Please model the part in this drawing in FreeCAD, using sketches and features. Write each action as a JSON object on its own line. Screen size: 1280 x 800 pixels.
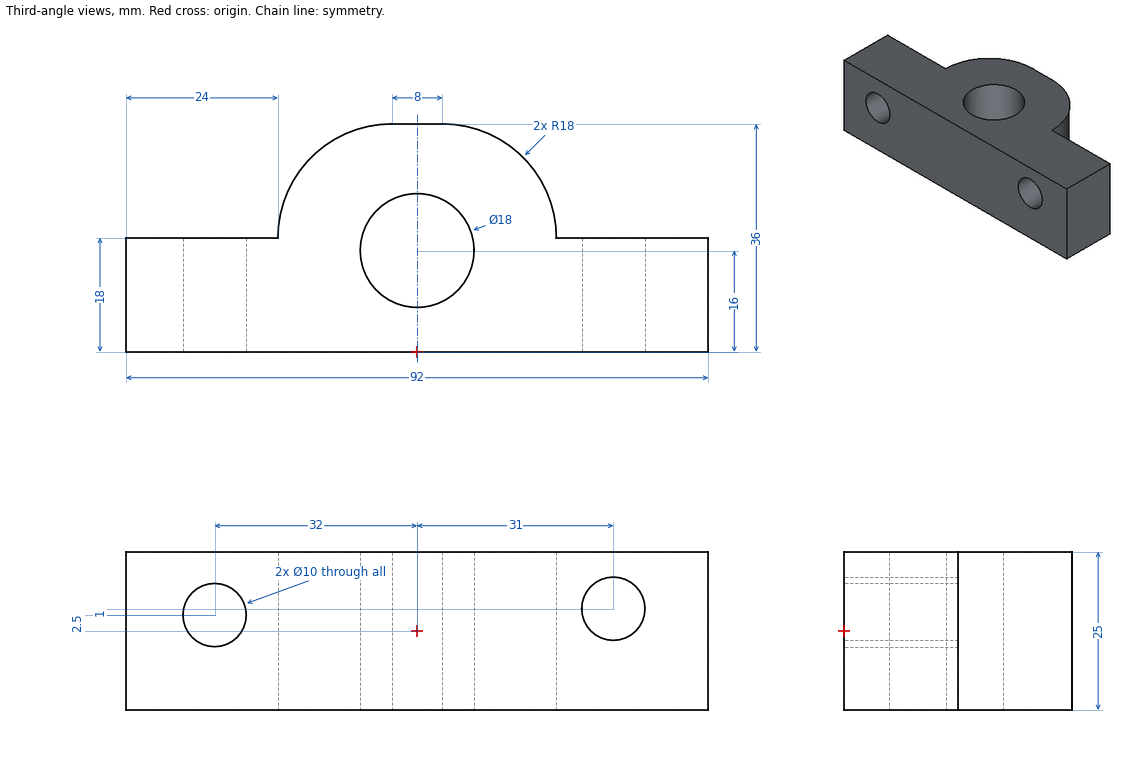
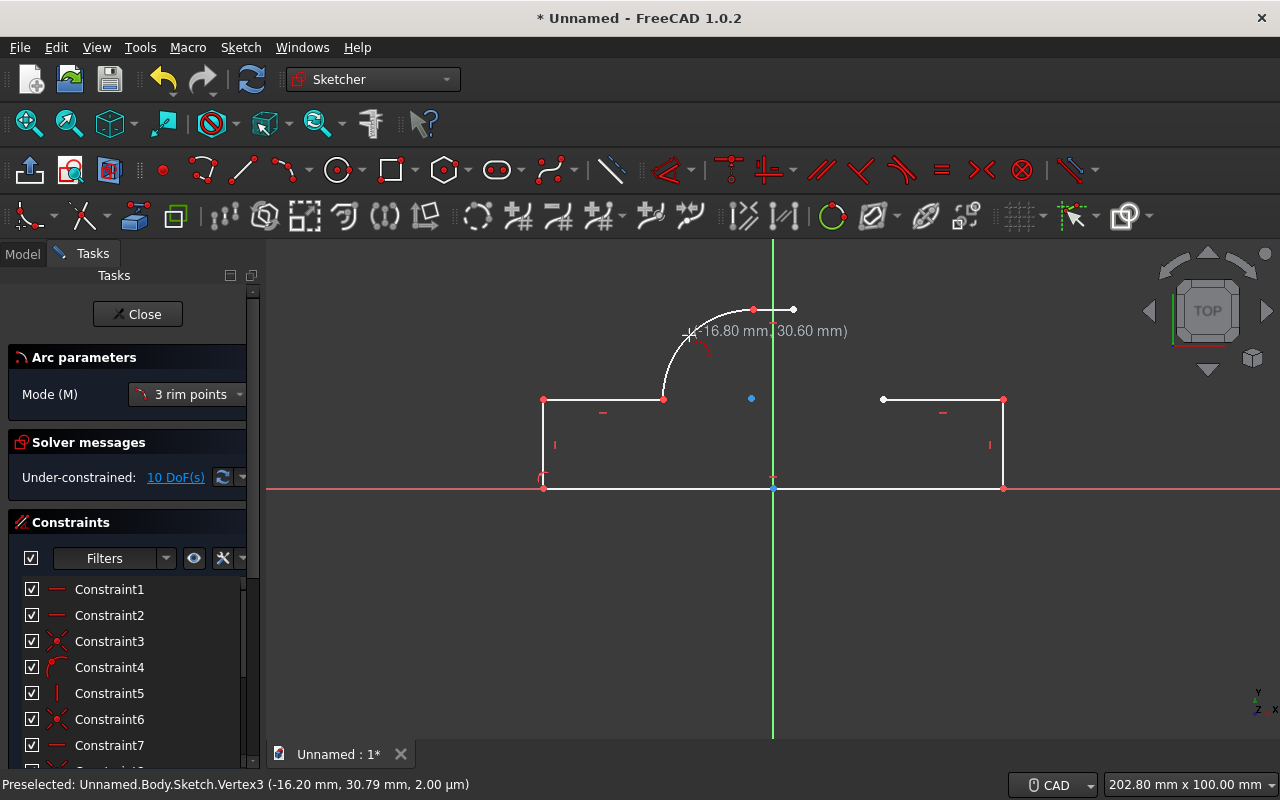
{"action": "left_click", "coordinate": [883, 400]}
{"action": "left_click", "coordinate": [793, 310]}
{"action": "left_click", "coordinate": [857, 335]}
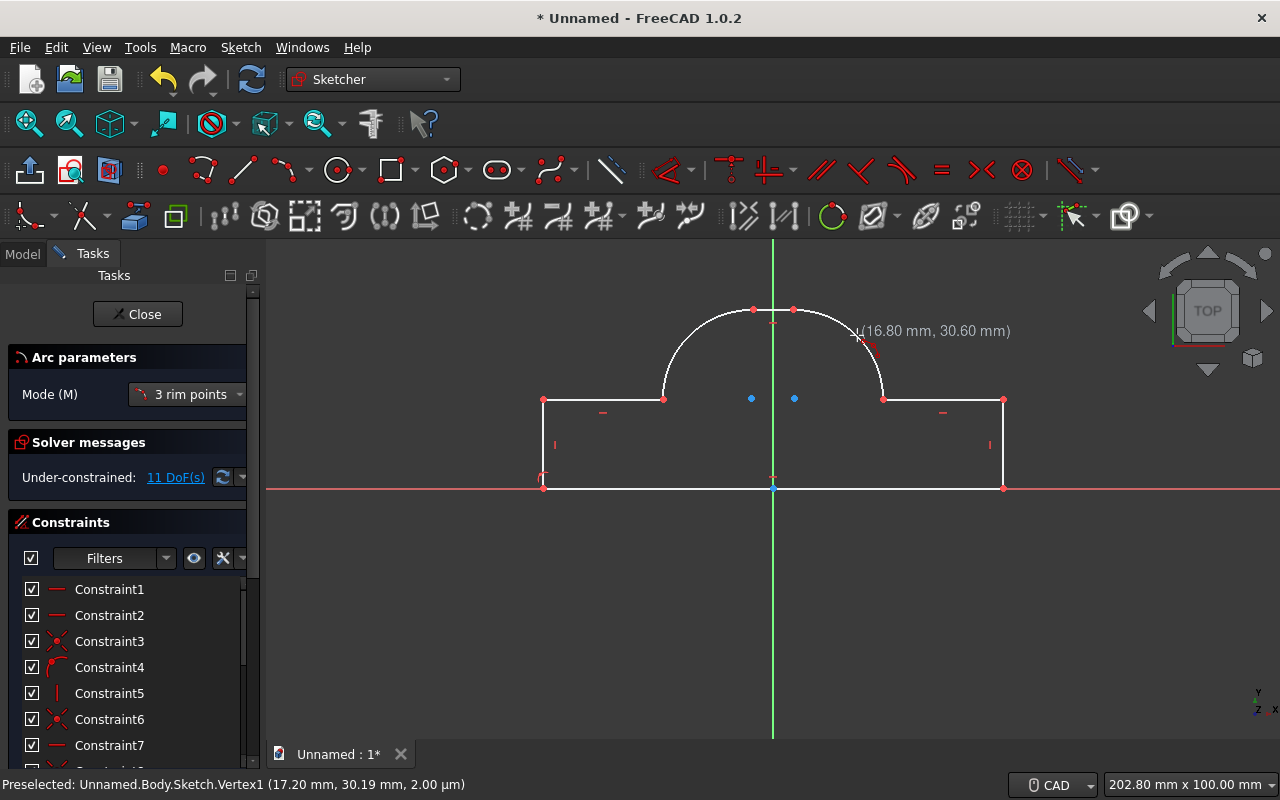
{"action": "left_click", "coordinate": [338, 170]}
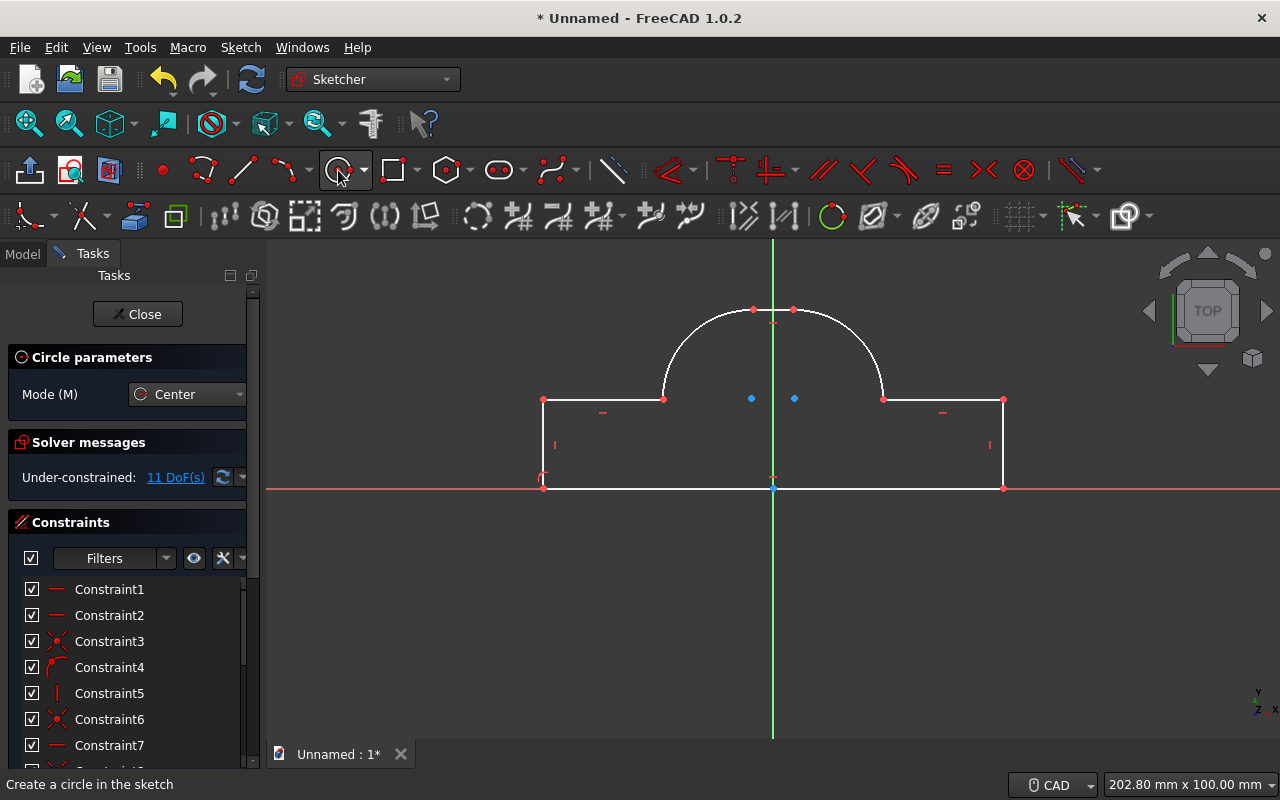
{"action": "left_click", "coordinate": [773, 409]}
{"action": "mouse_move", "coordinate": [805, 377]}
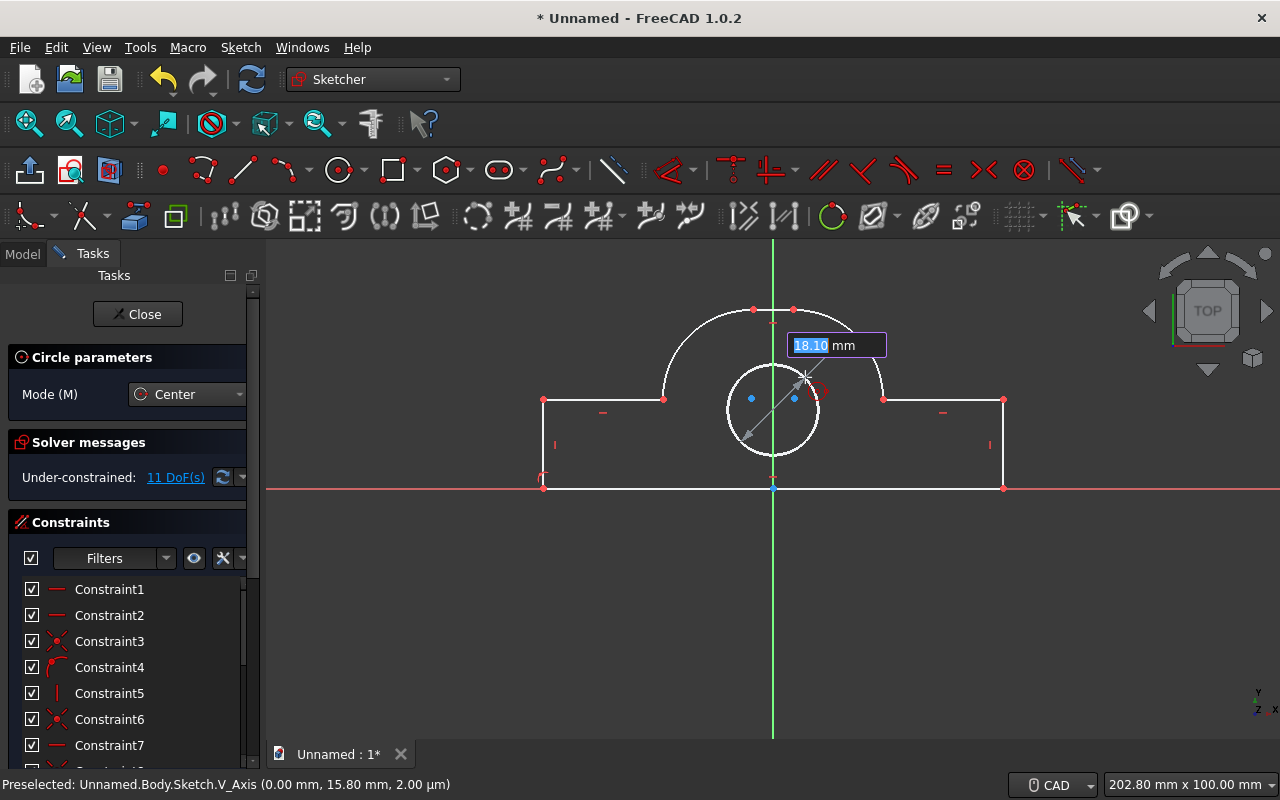
{"action": "type", "text": "18"}
{"action": "key", "text": "Return"}
{"action": "key", "text": "Escape"}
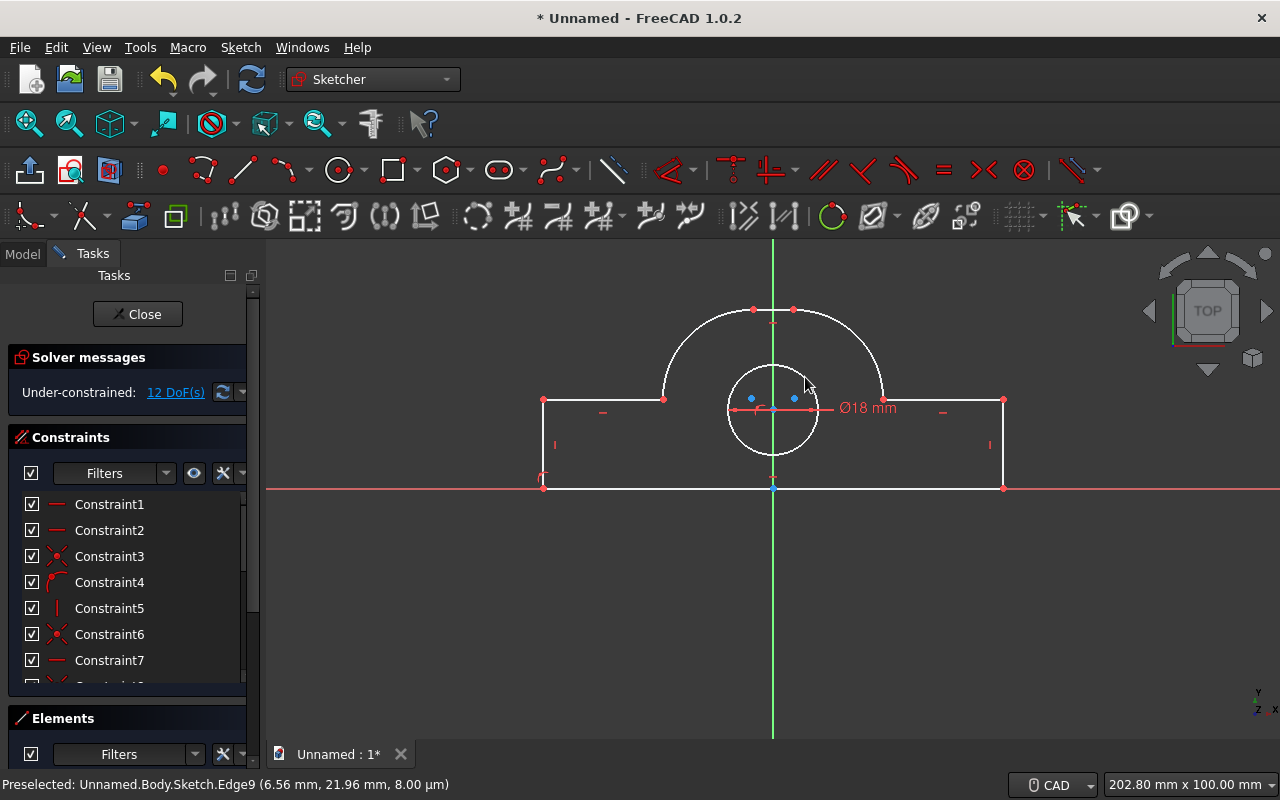
{"action": "left_click", "coordinate": [773, 310]}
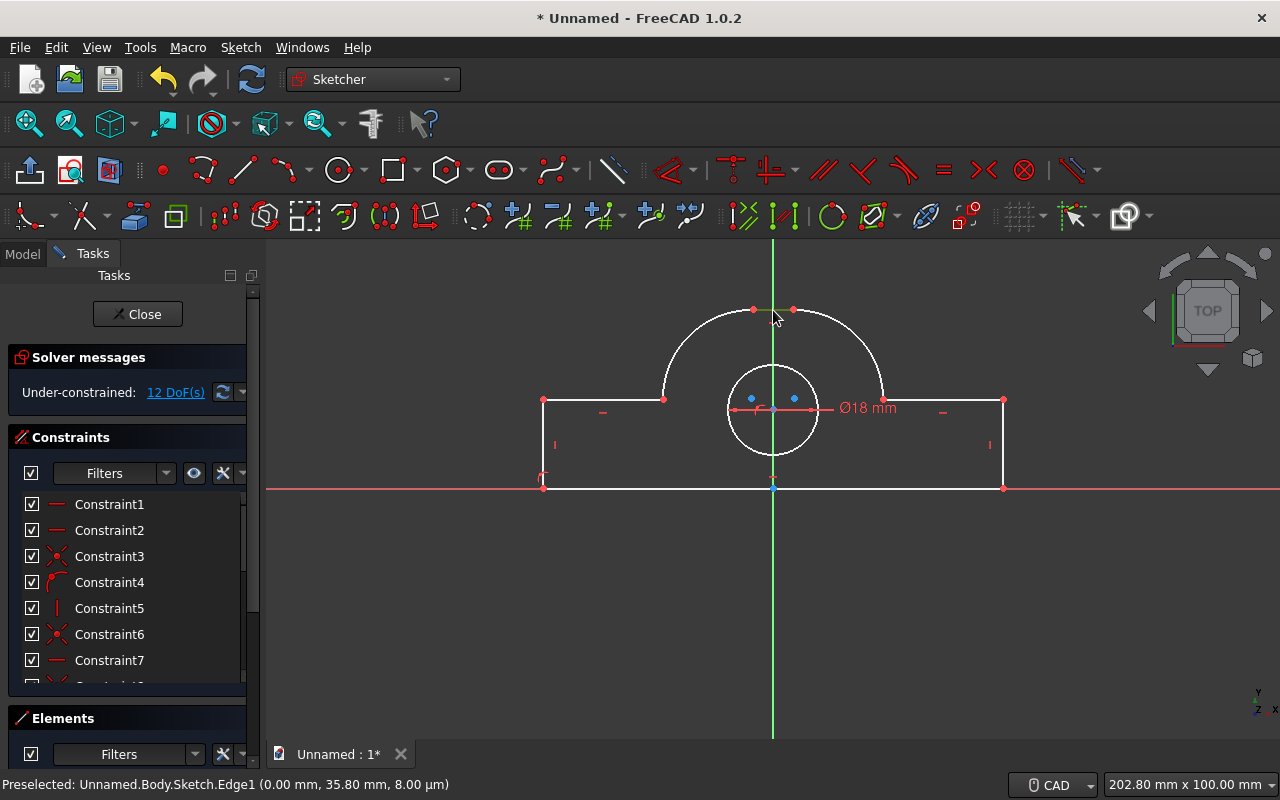
{"action": "left_click", "coordinate": [712, 319]}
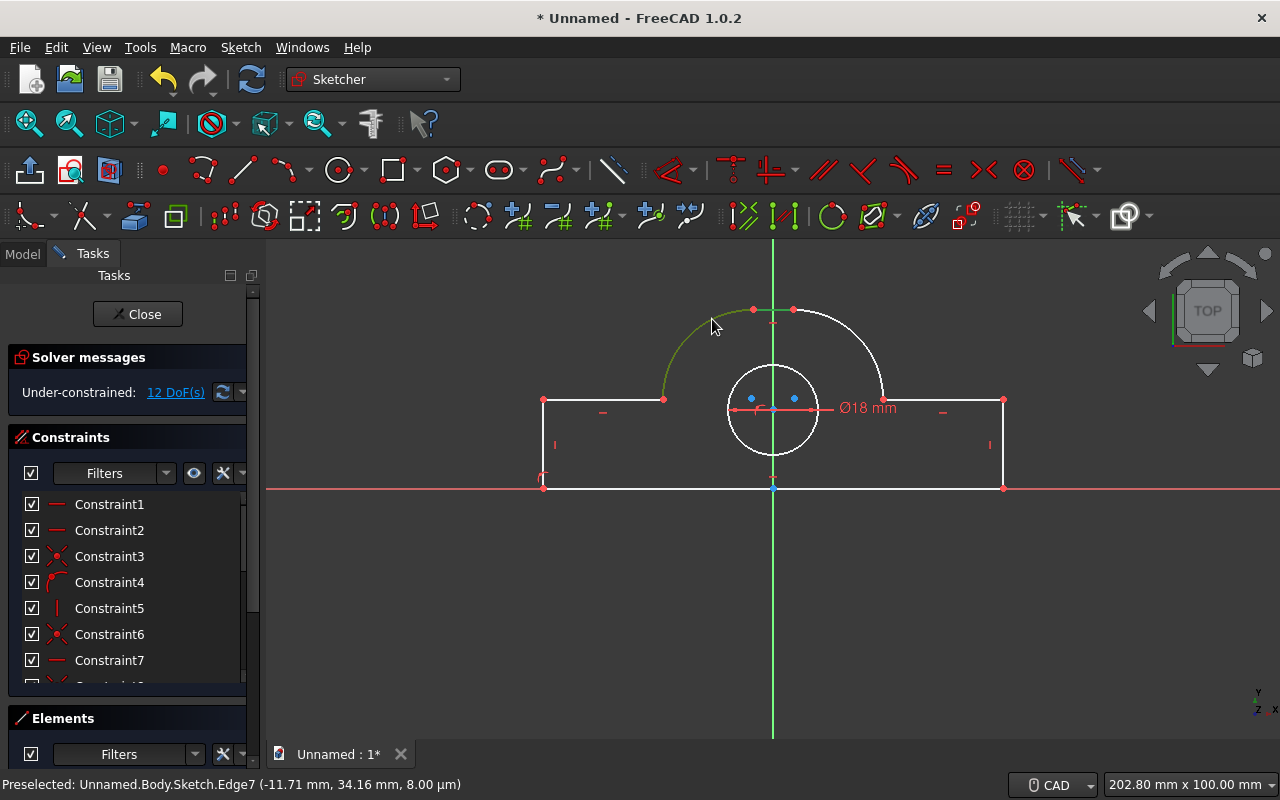
{"action": "left_click", "coordinate": [904, 170]}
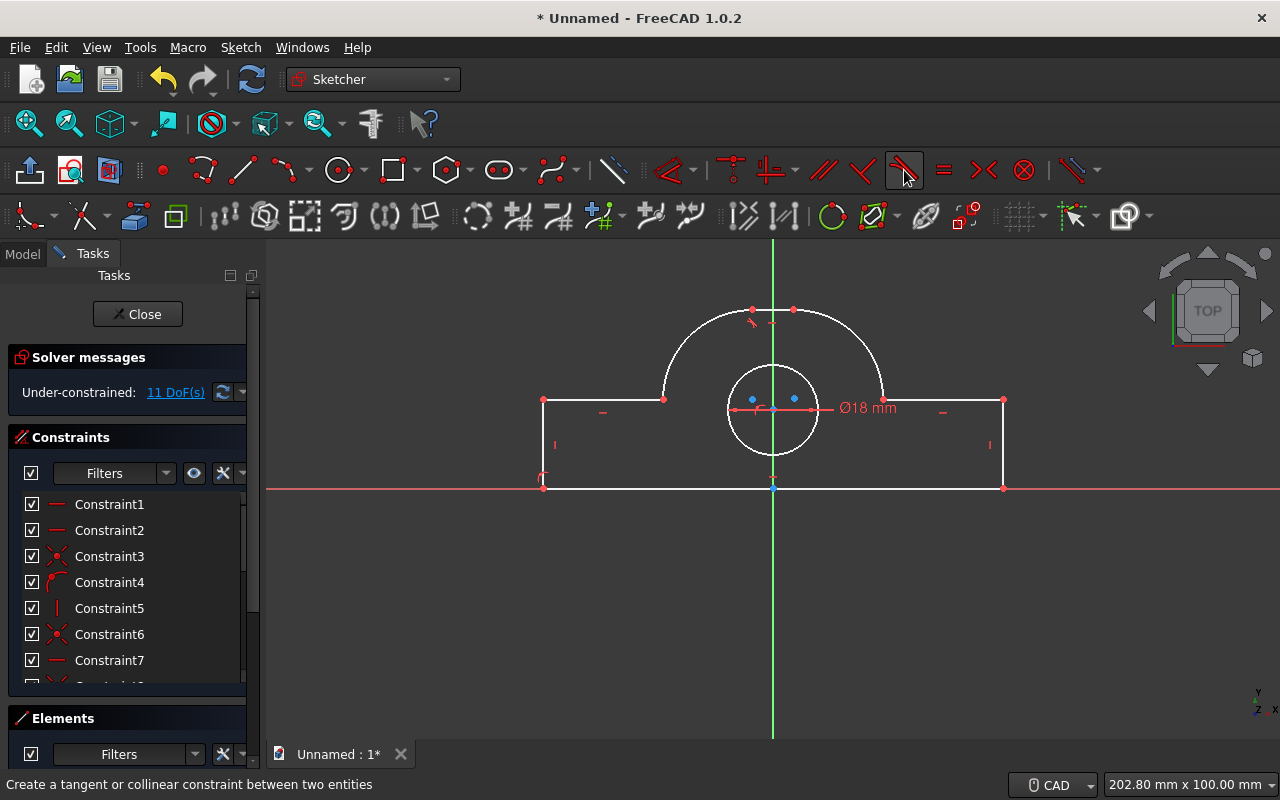
{"action": "left_click", "coordinate": [777, 310]}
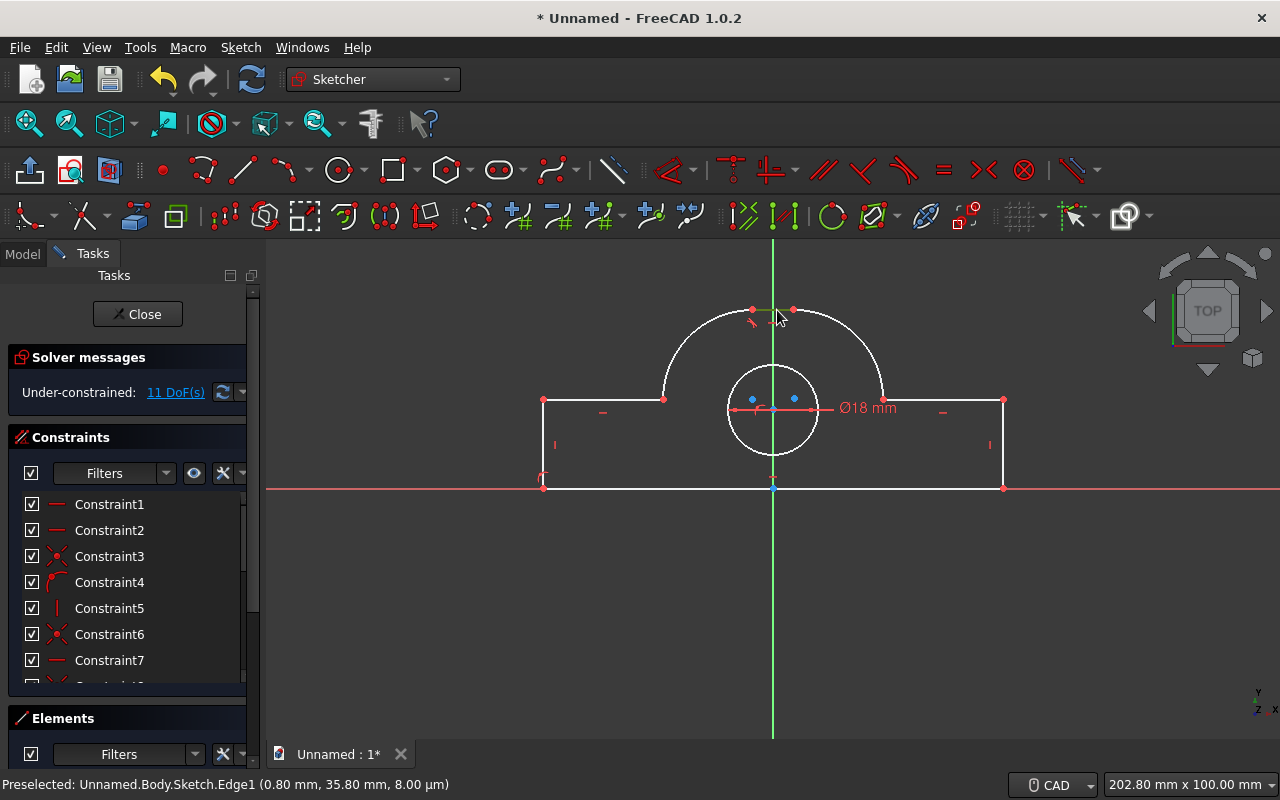
{"action": "left_click", "coordinate": [874, 359]}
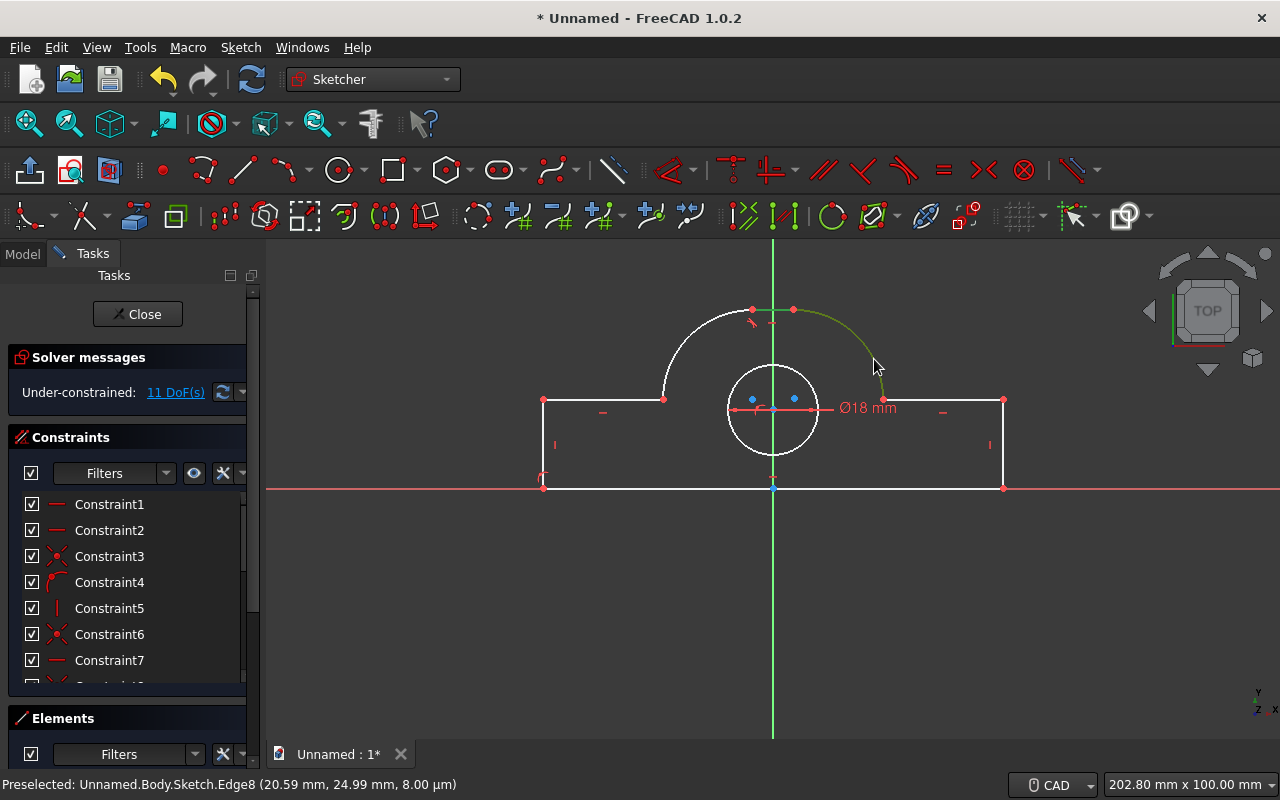
{"action": "left_click", "coordinate": [904, 170]}